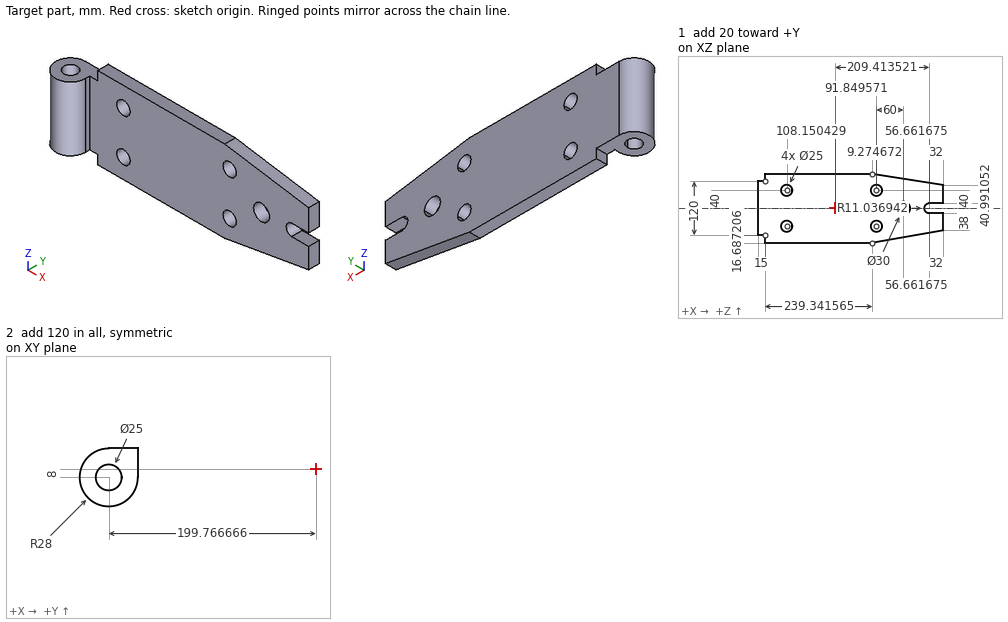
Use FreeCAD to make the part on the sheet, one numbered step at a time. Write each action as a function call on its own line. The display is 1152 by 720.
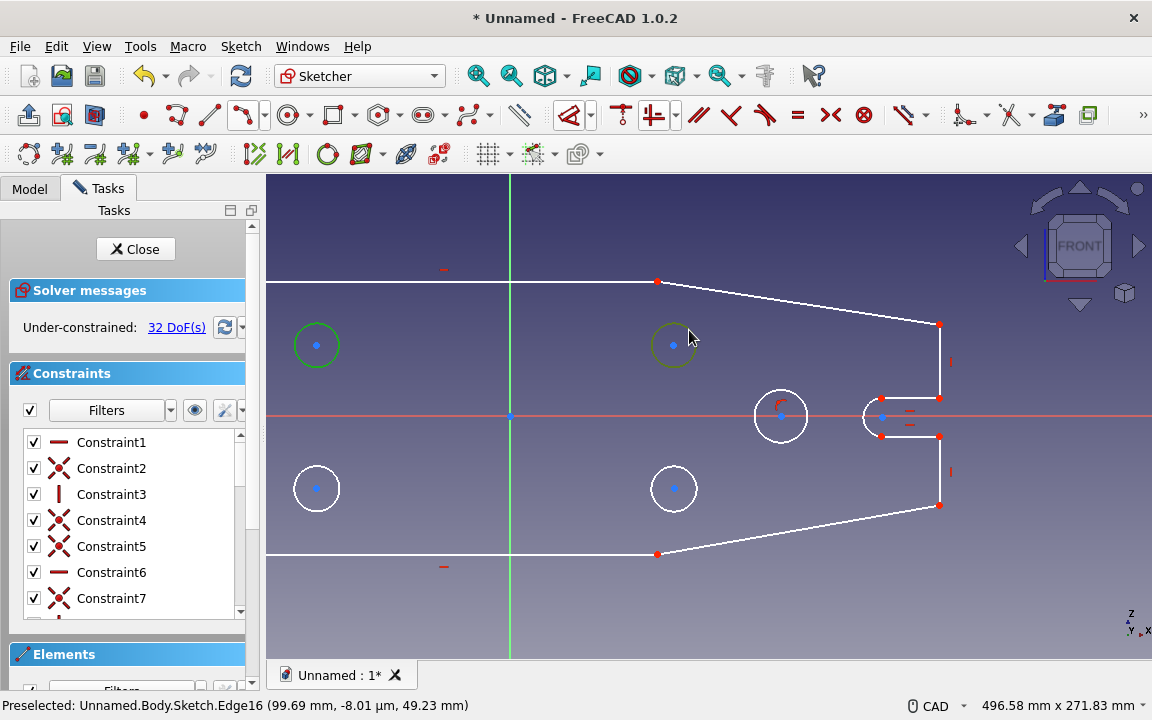
click(333, 473)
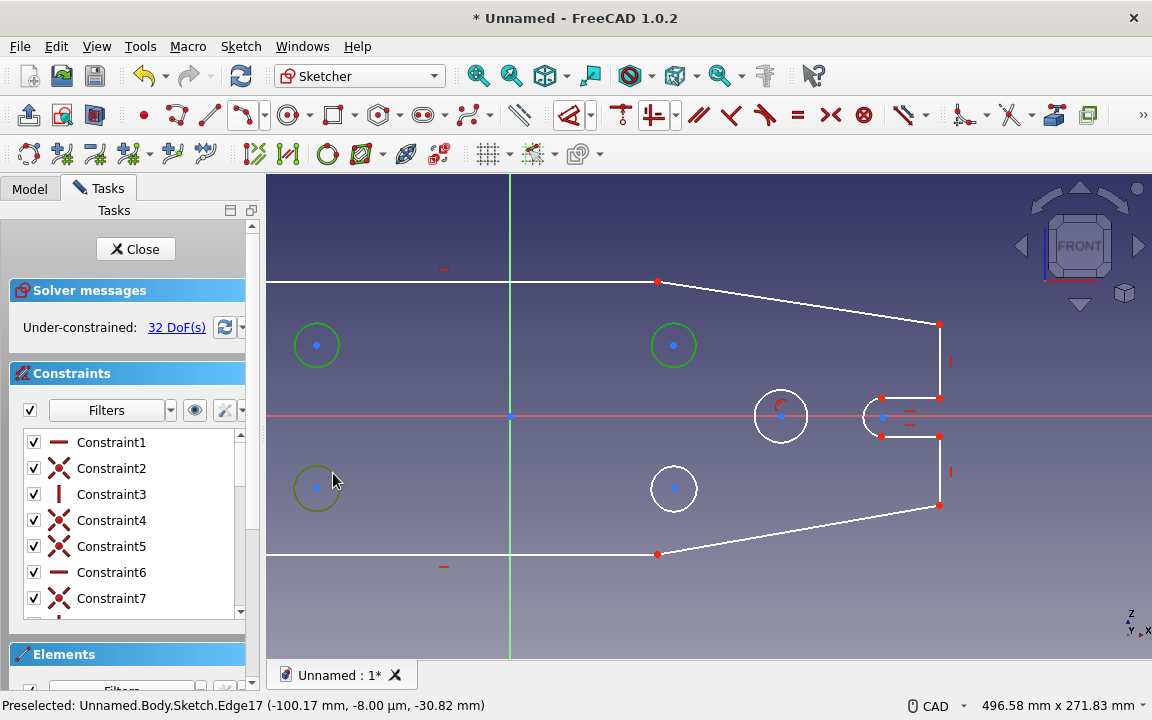
click(690, 473)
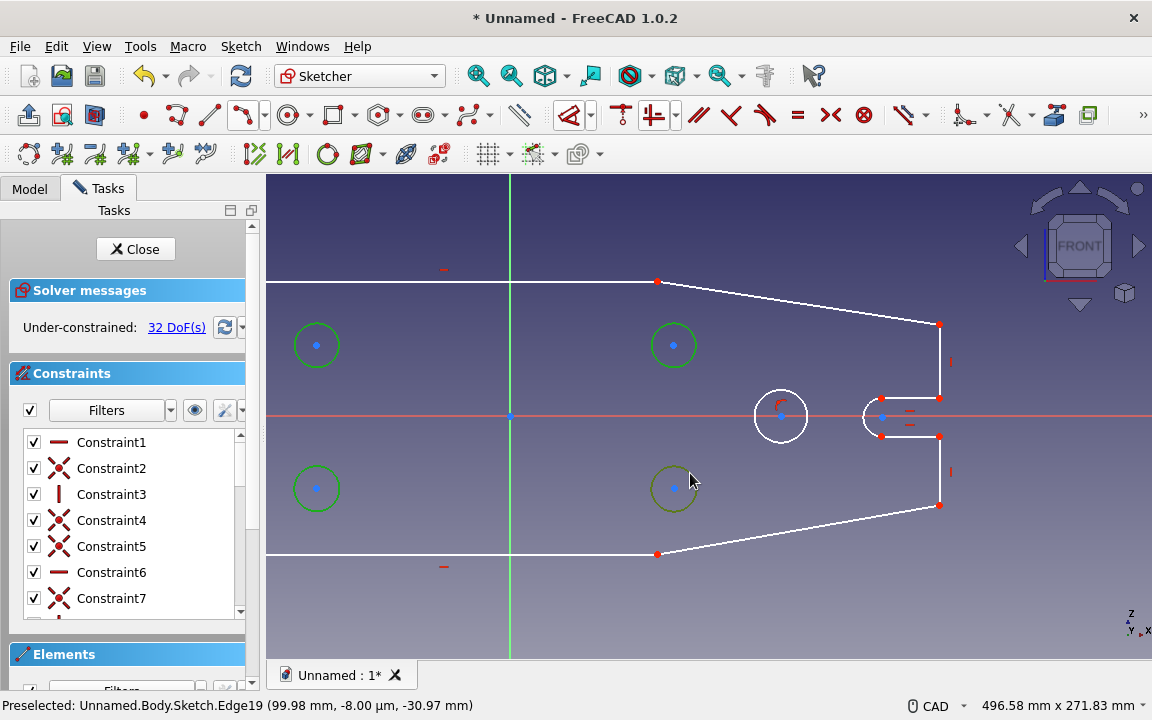
click(798, 116)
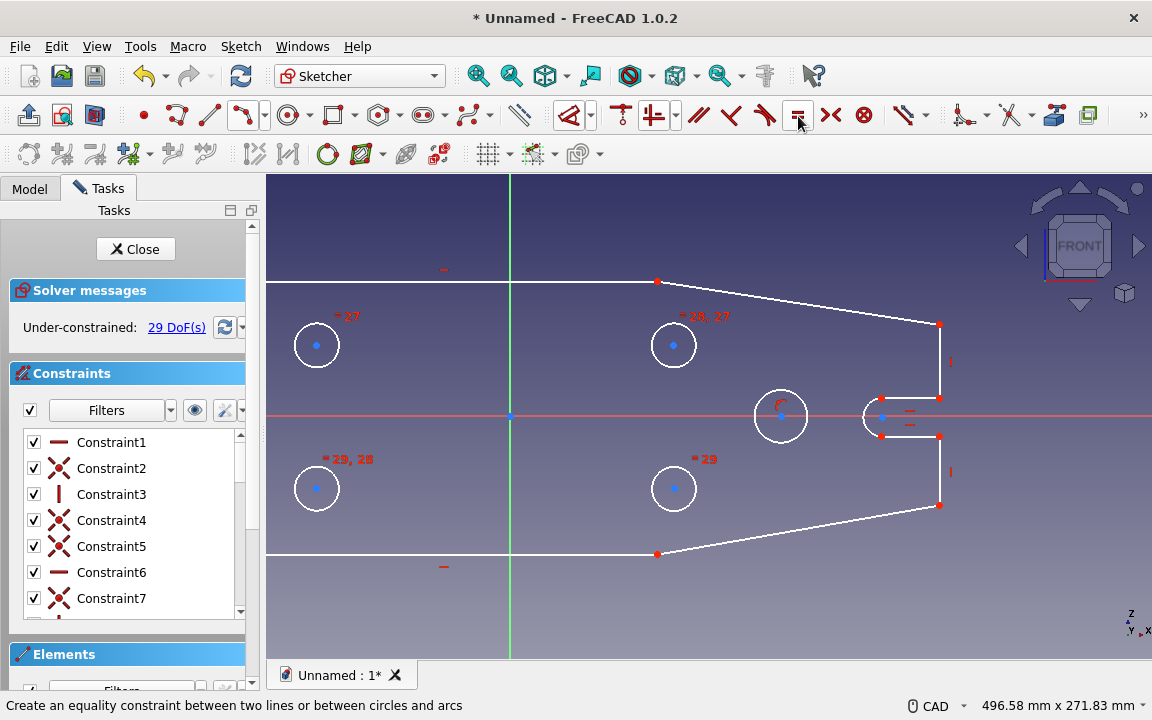
click(883, 417)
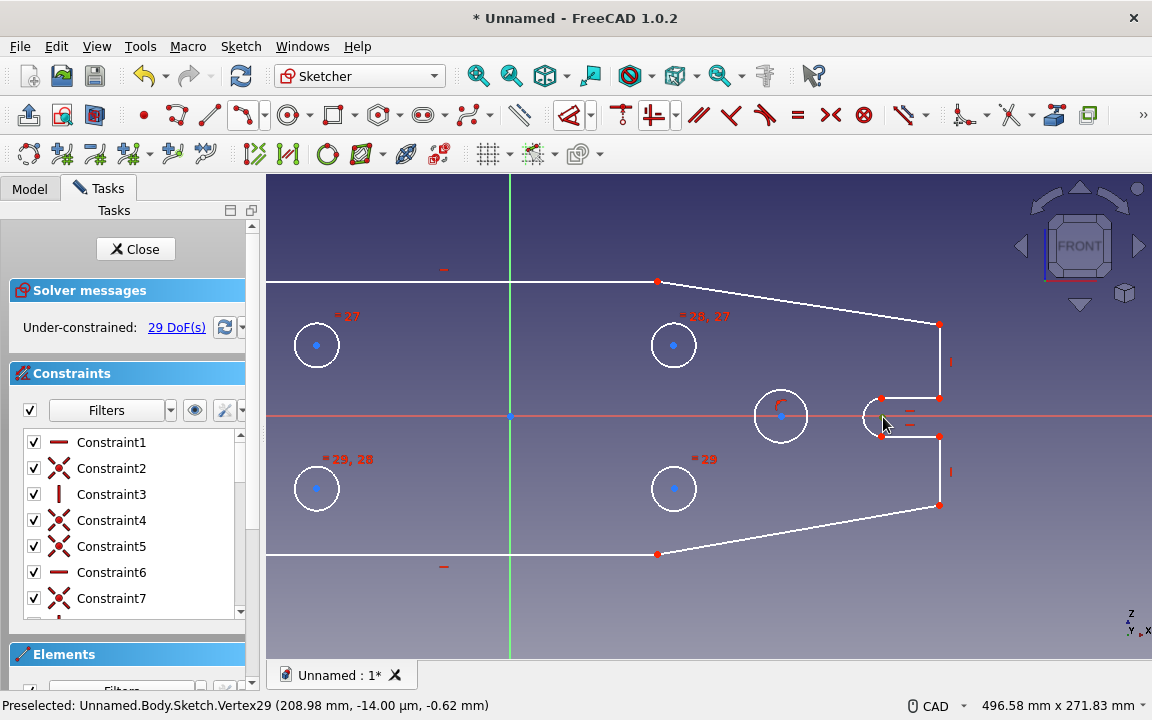
click(344, 416)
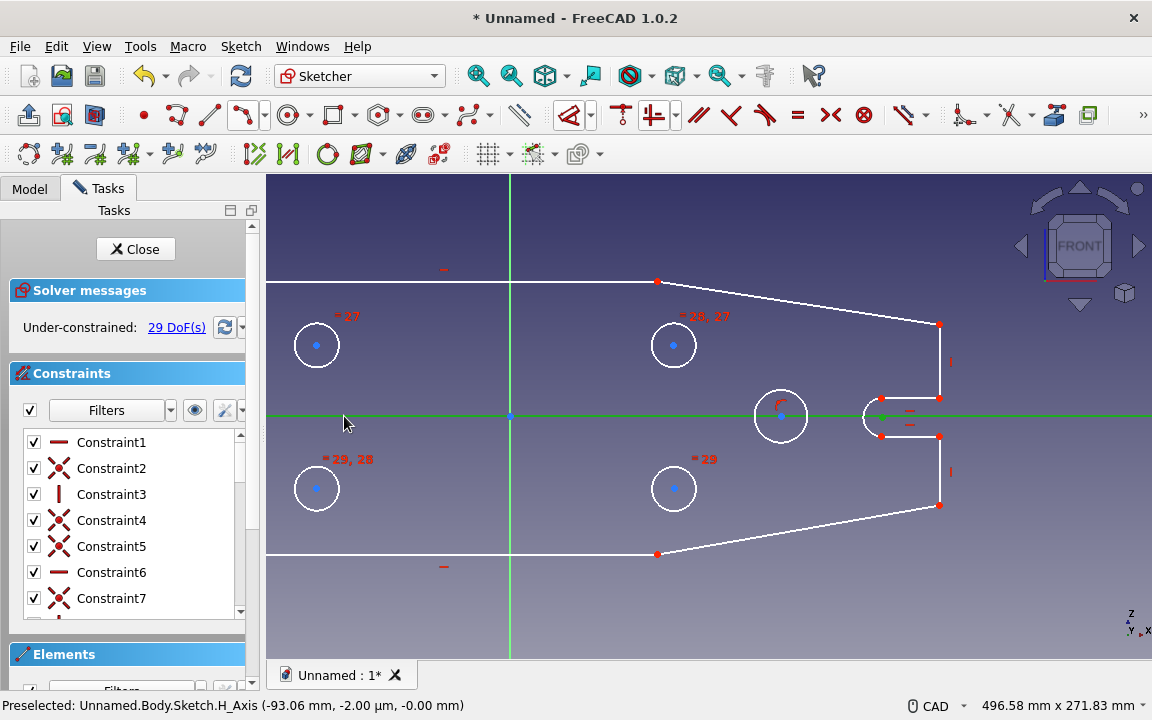
click(621, 116)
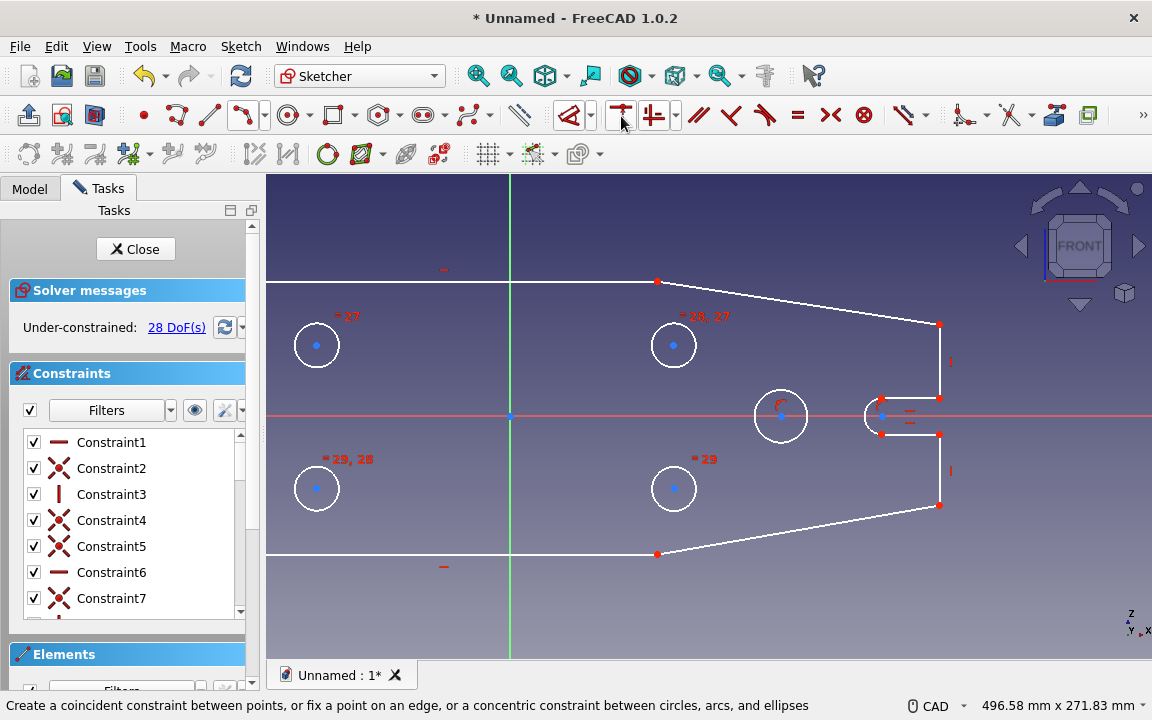
click(317, 345)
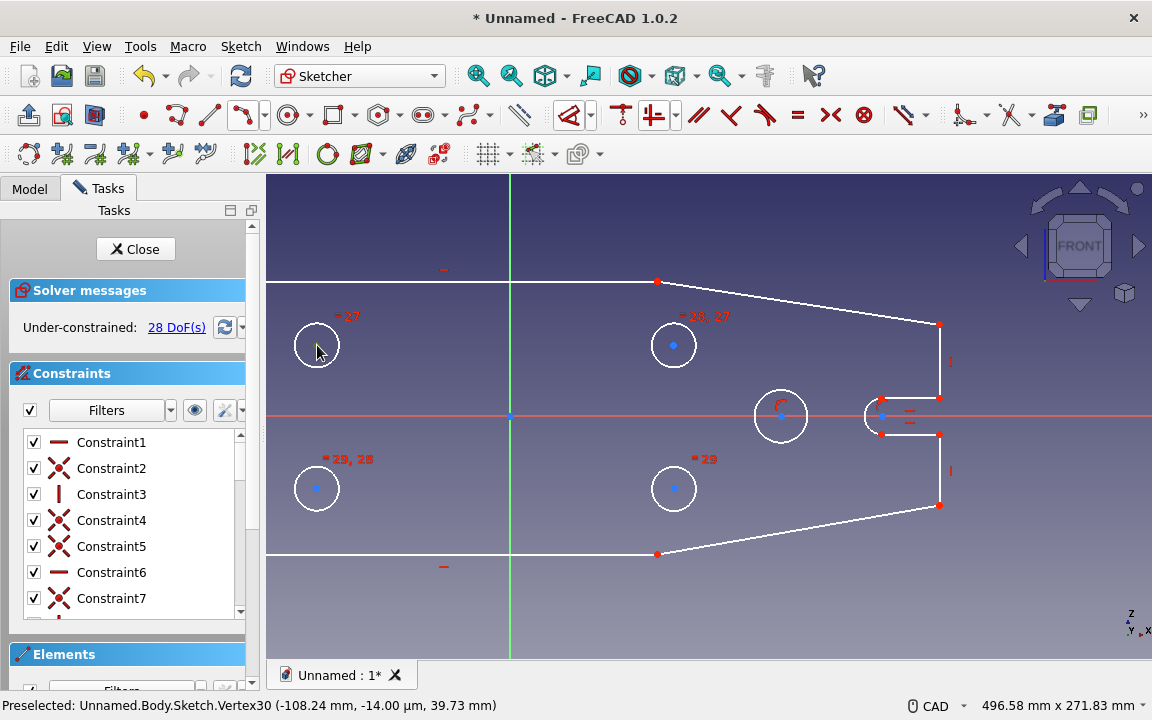
click(317, 489)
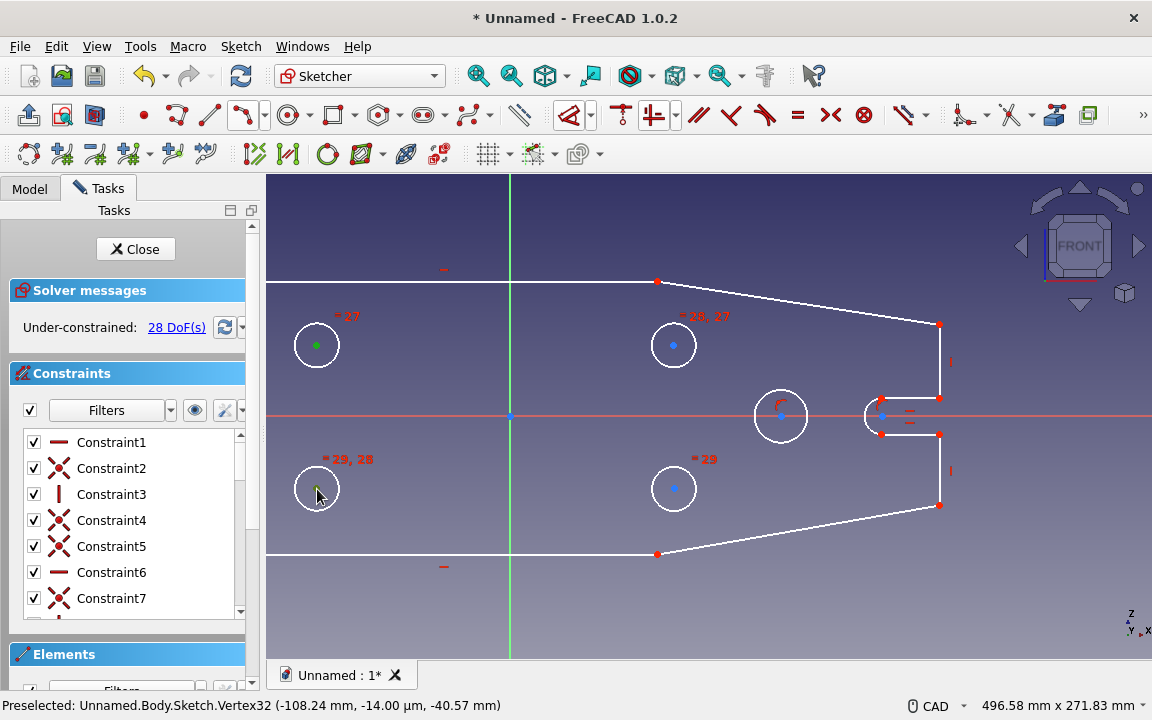
click(344, 416)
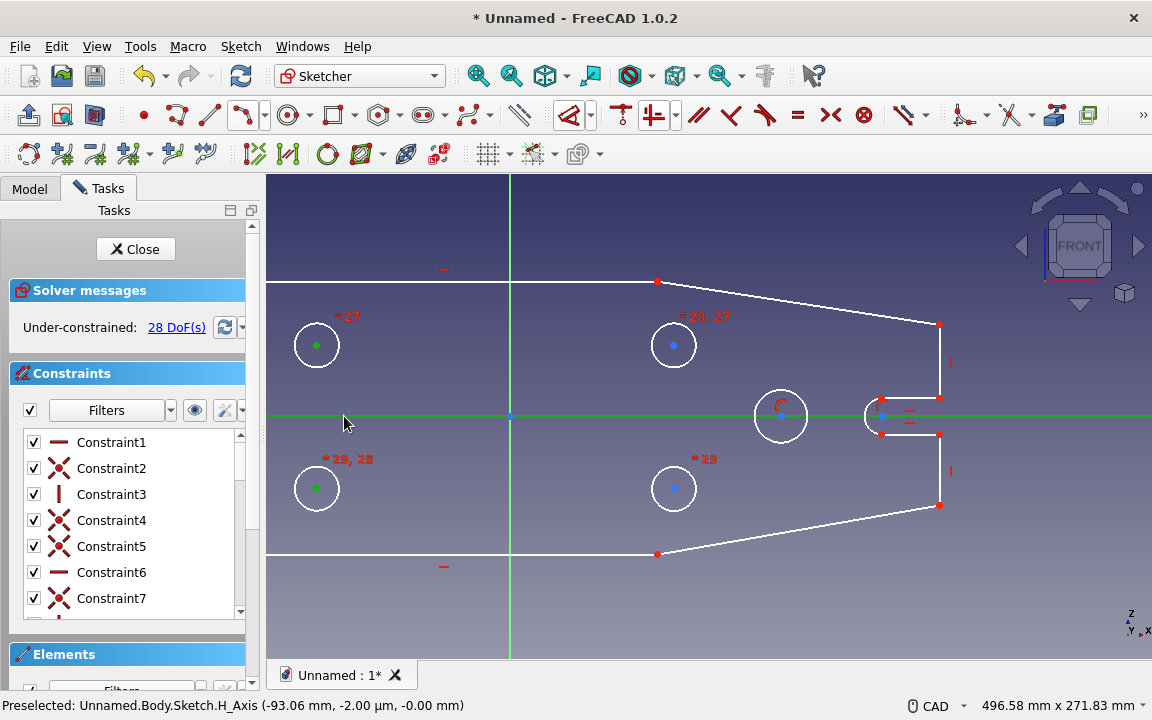
click(831, 116)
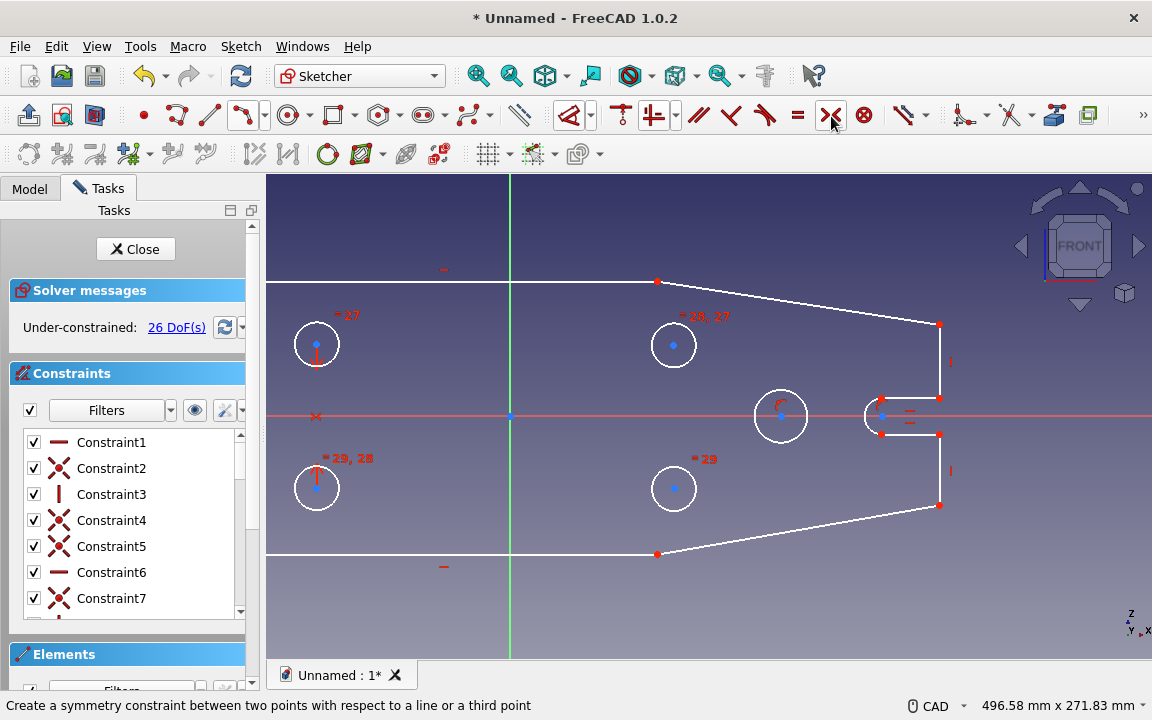
click(674, 345)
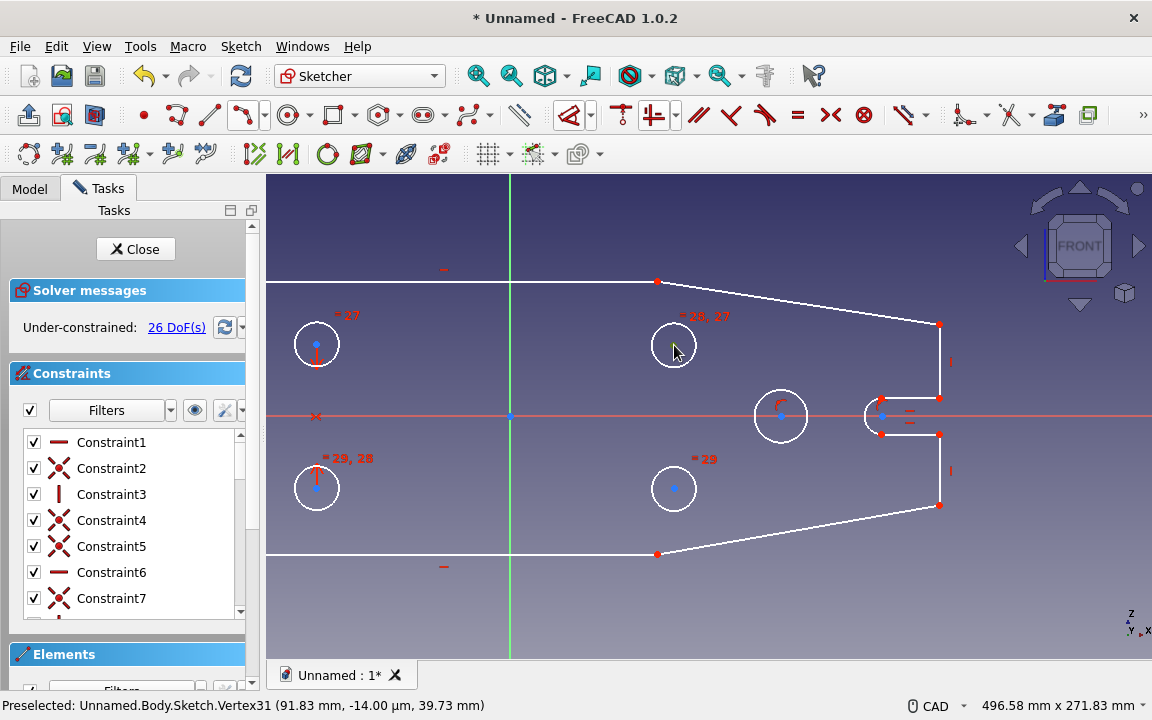
click(674, 489)